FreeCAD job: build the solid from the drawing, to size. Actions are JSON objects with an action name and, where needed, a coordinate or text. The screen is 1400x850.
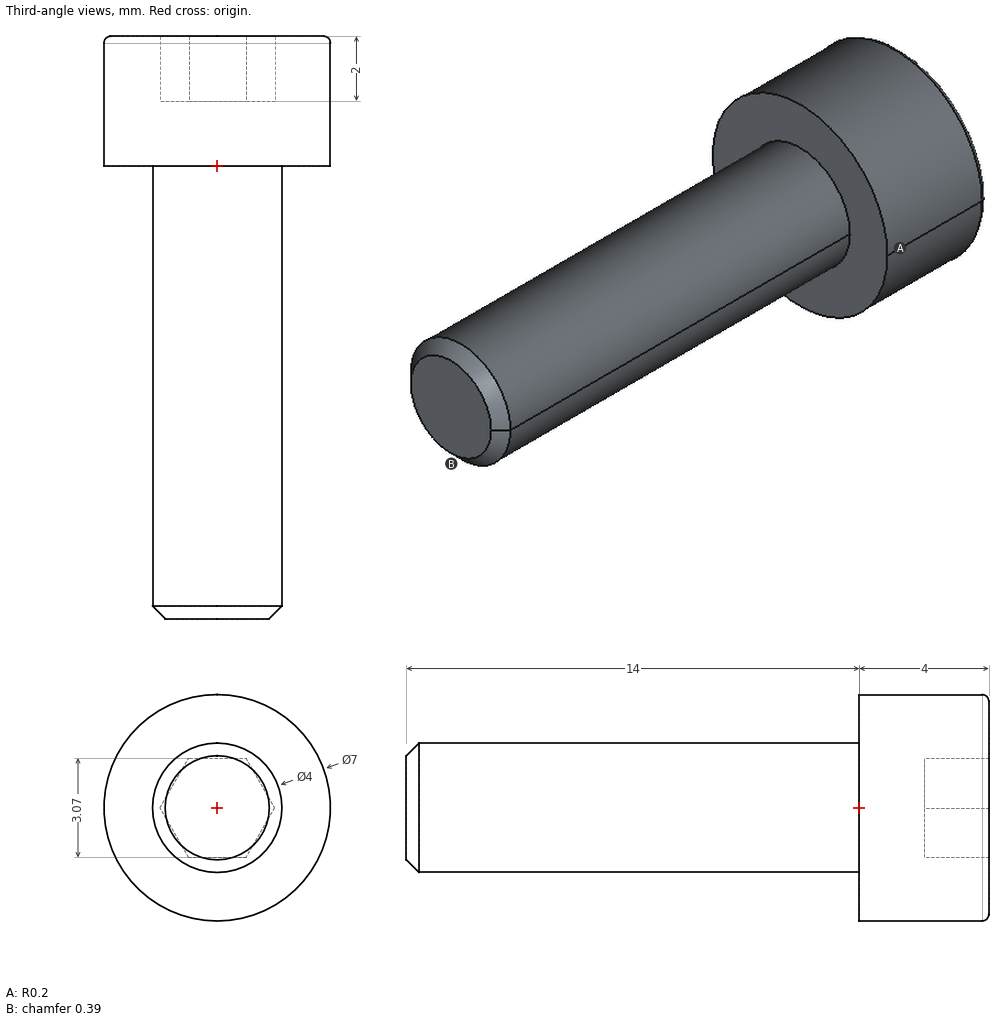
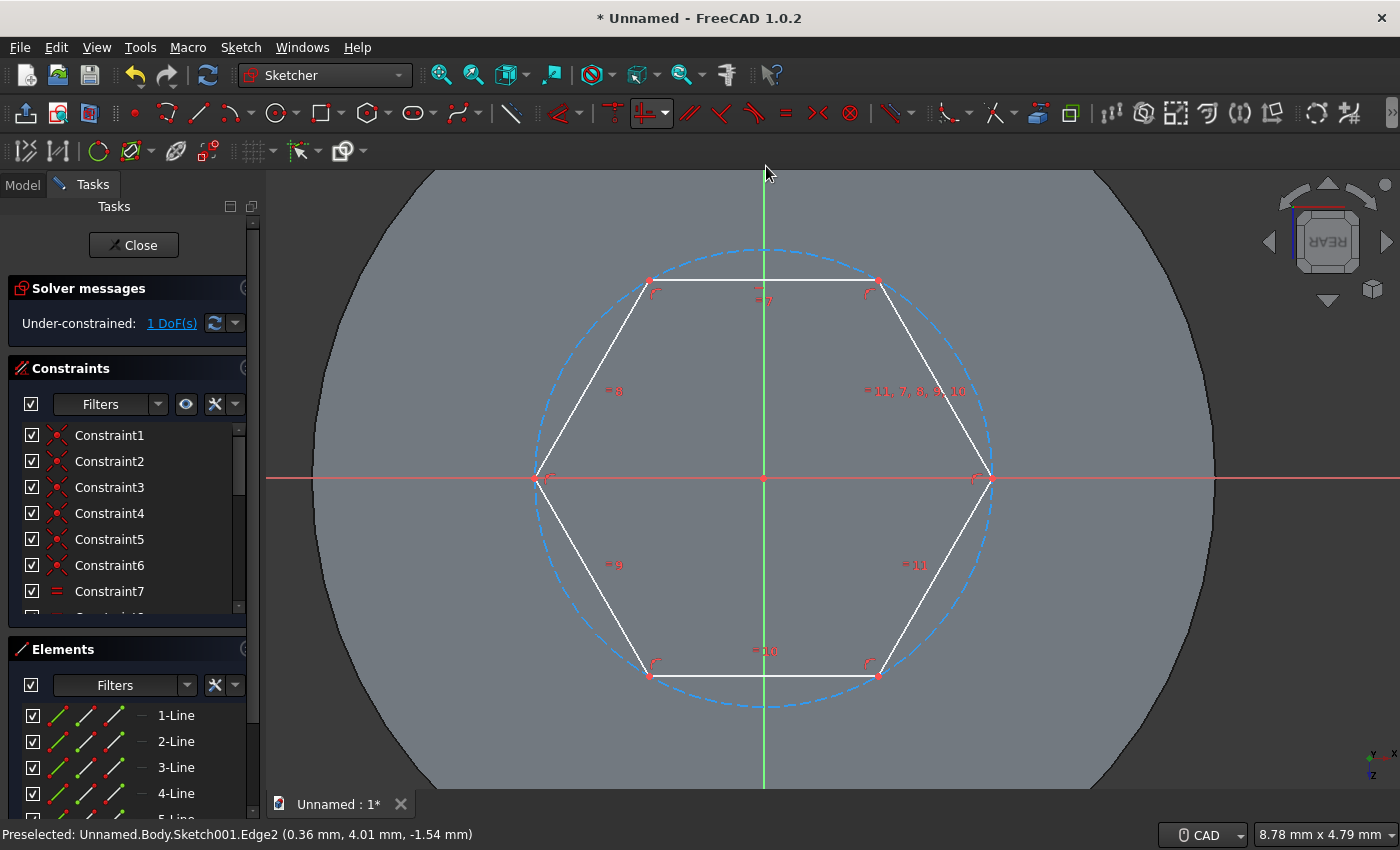
{"action": "left_click", "coordinate": [558, 114]}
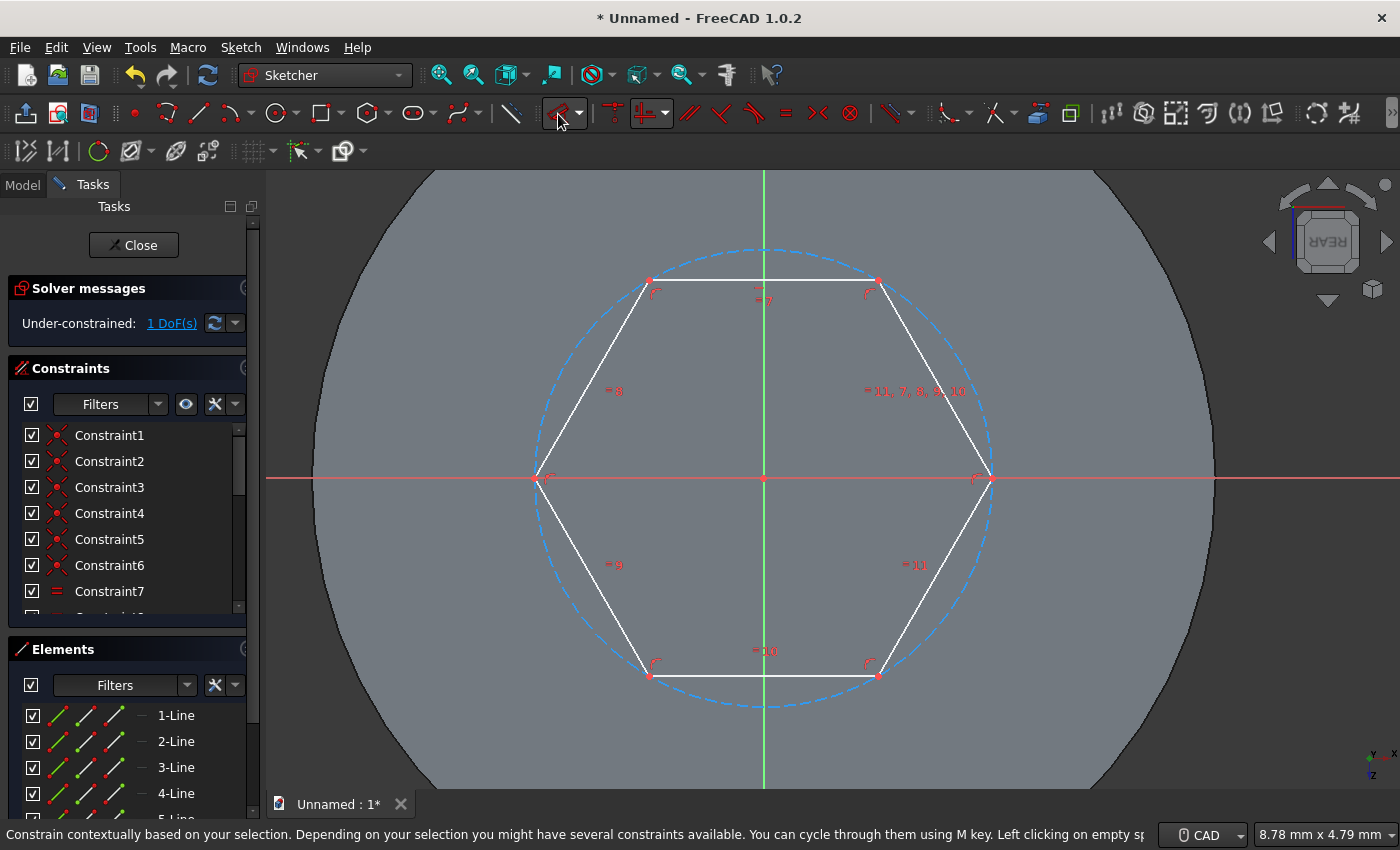
{"action": "left_click", "coordinate": [649, 676]}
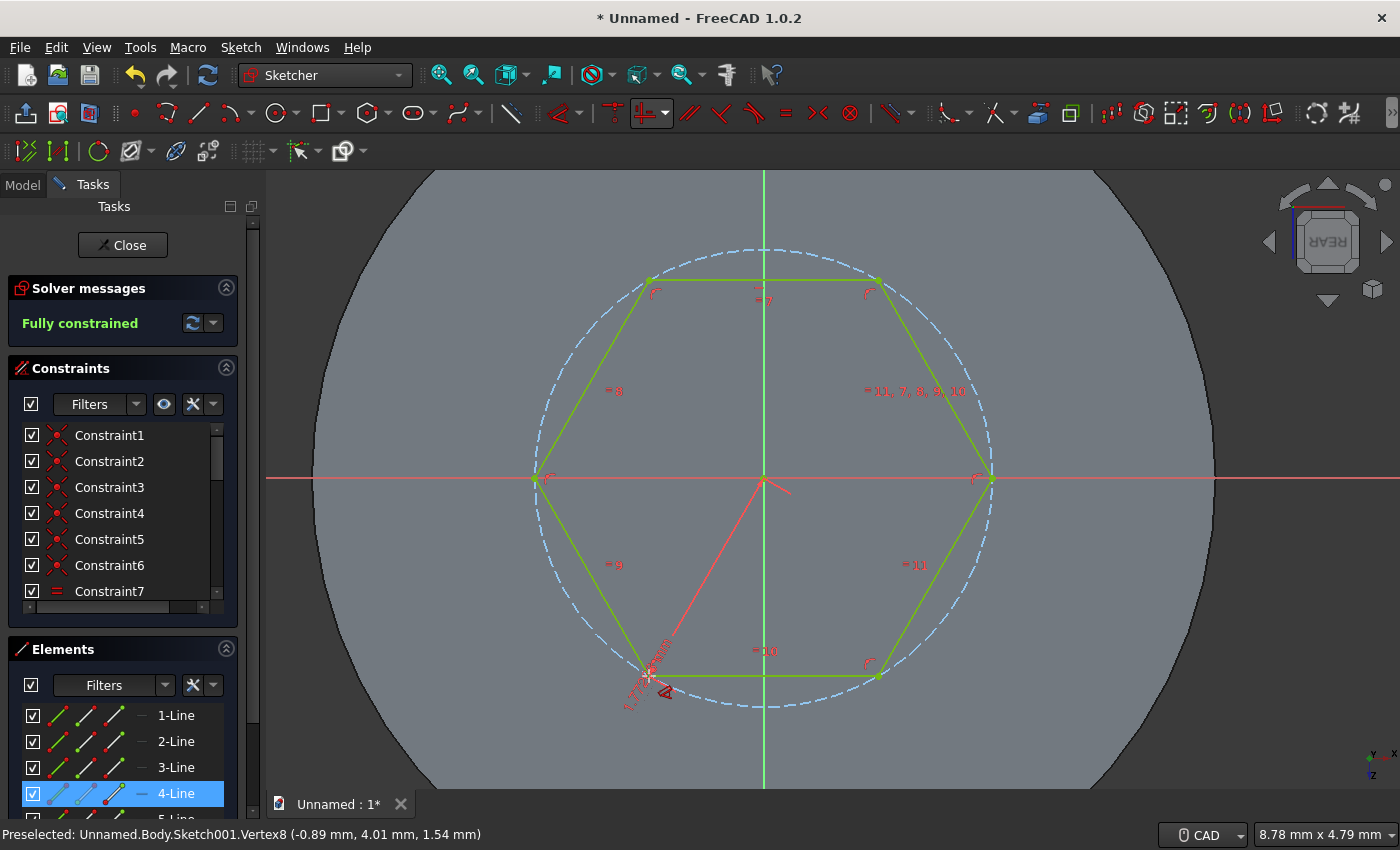
{"action": "left_click", "coordinate": [878, 280]}
{"action": "left_click", "coordinate": [615, 387]}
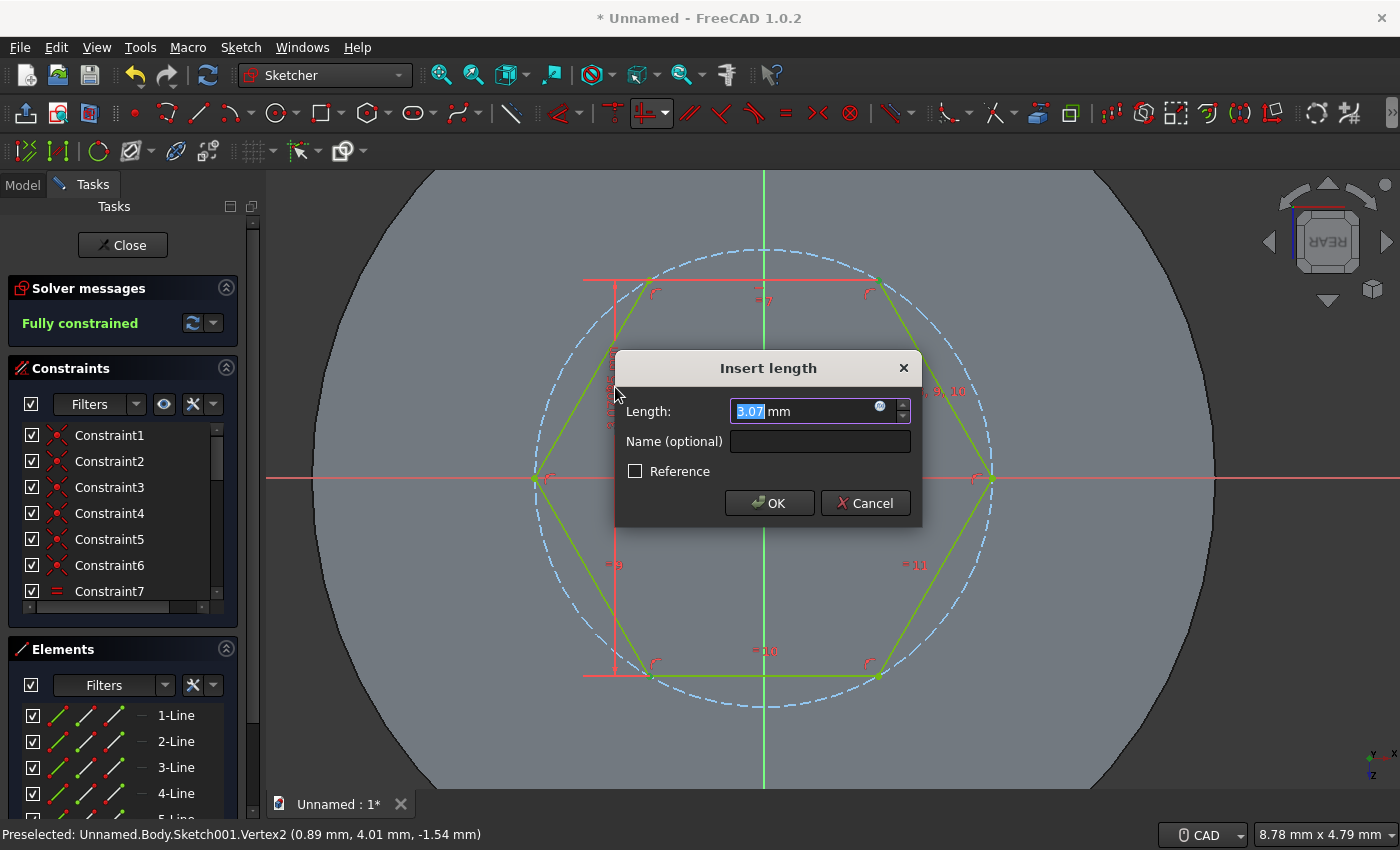
{"action": "type", "text": "3.07"}
{"action": "key", "text": "Return"}
{"action": "key", "text": "Escape"}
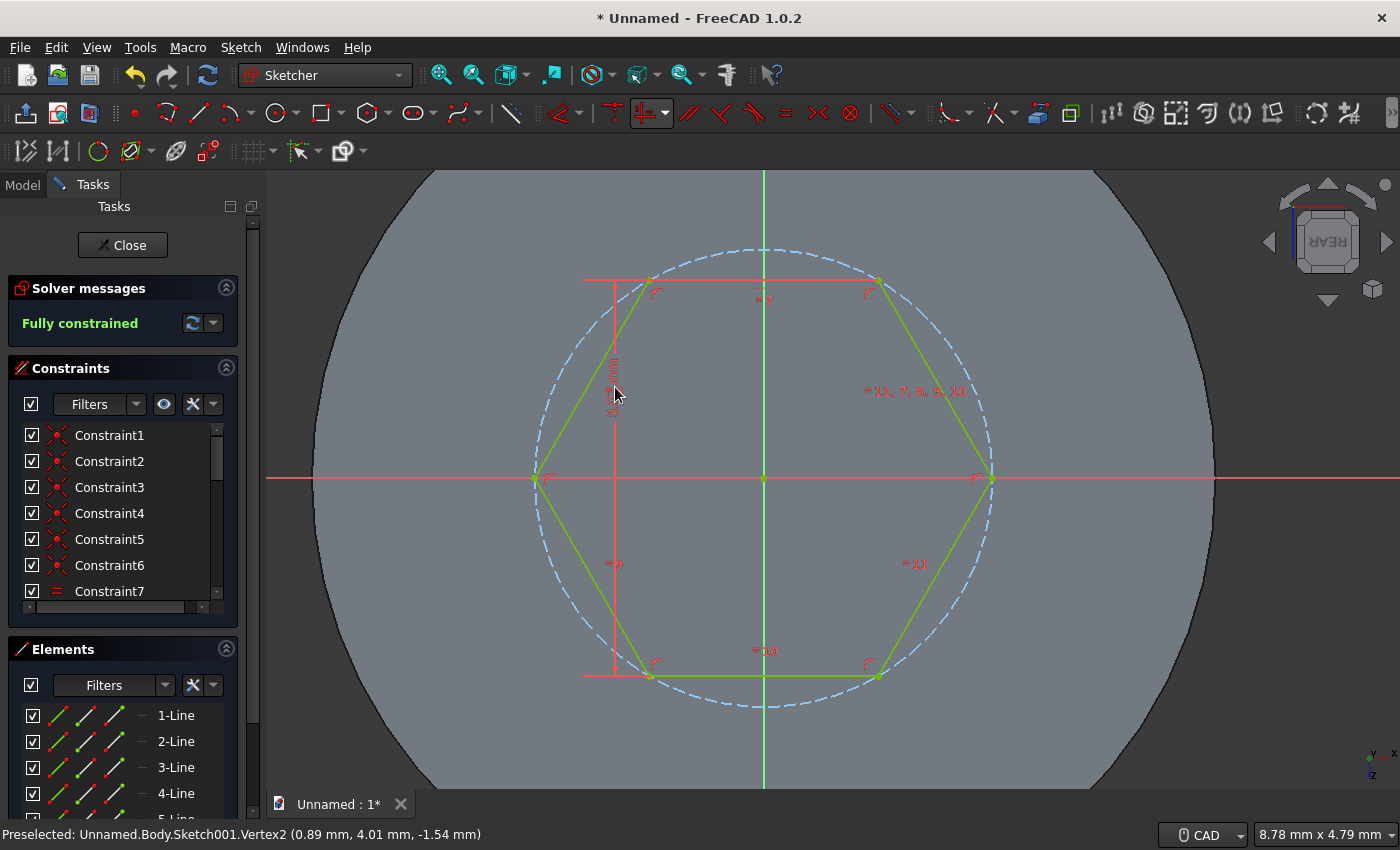
{"action": "left_click", "coordinate": [123, 245]}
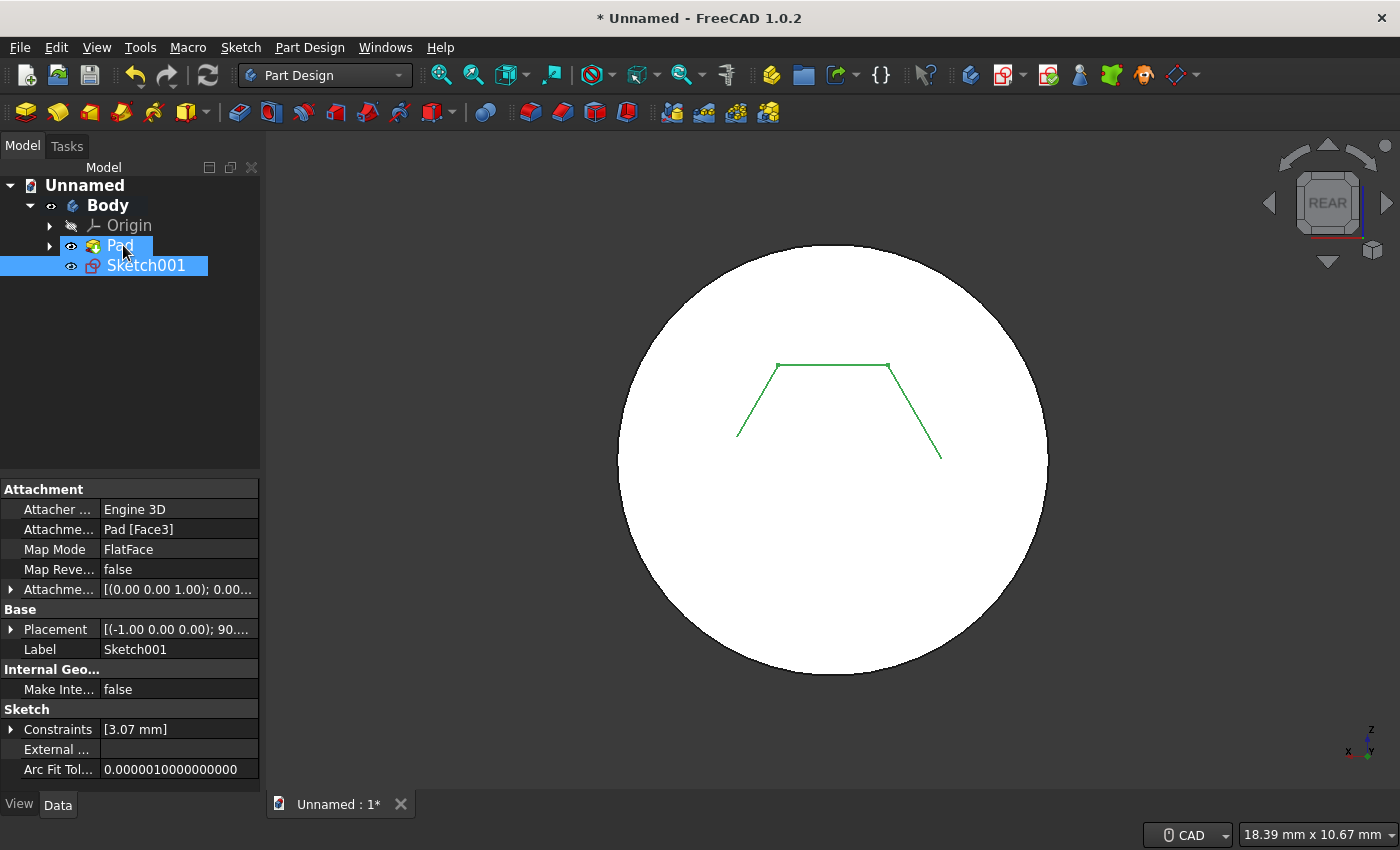
{"action": "left_click", "coordinate": [240, 112]}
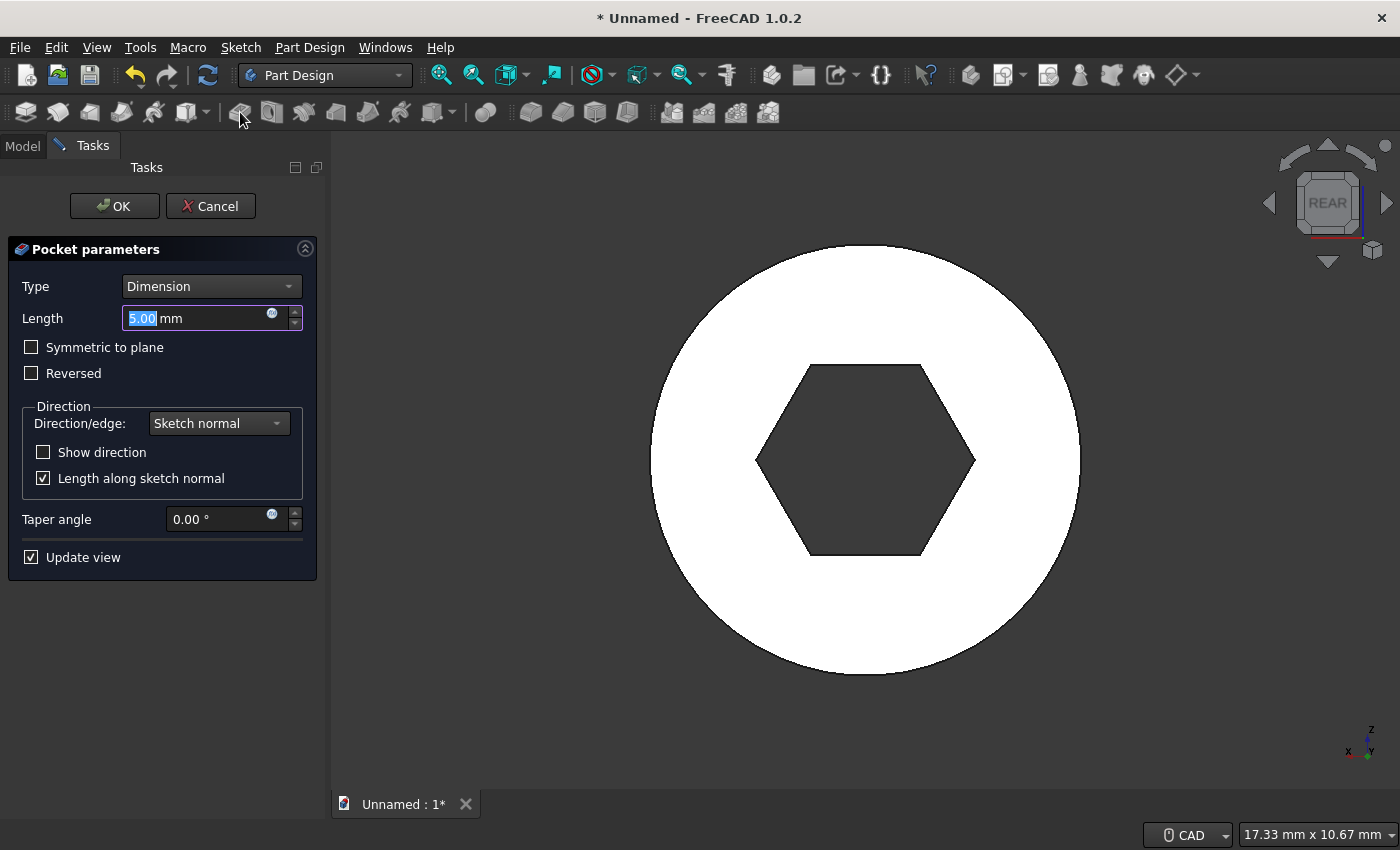
{"action": "type", "text": "2"}
{"action": "key", "text": "Tab"}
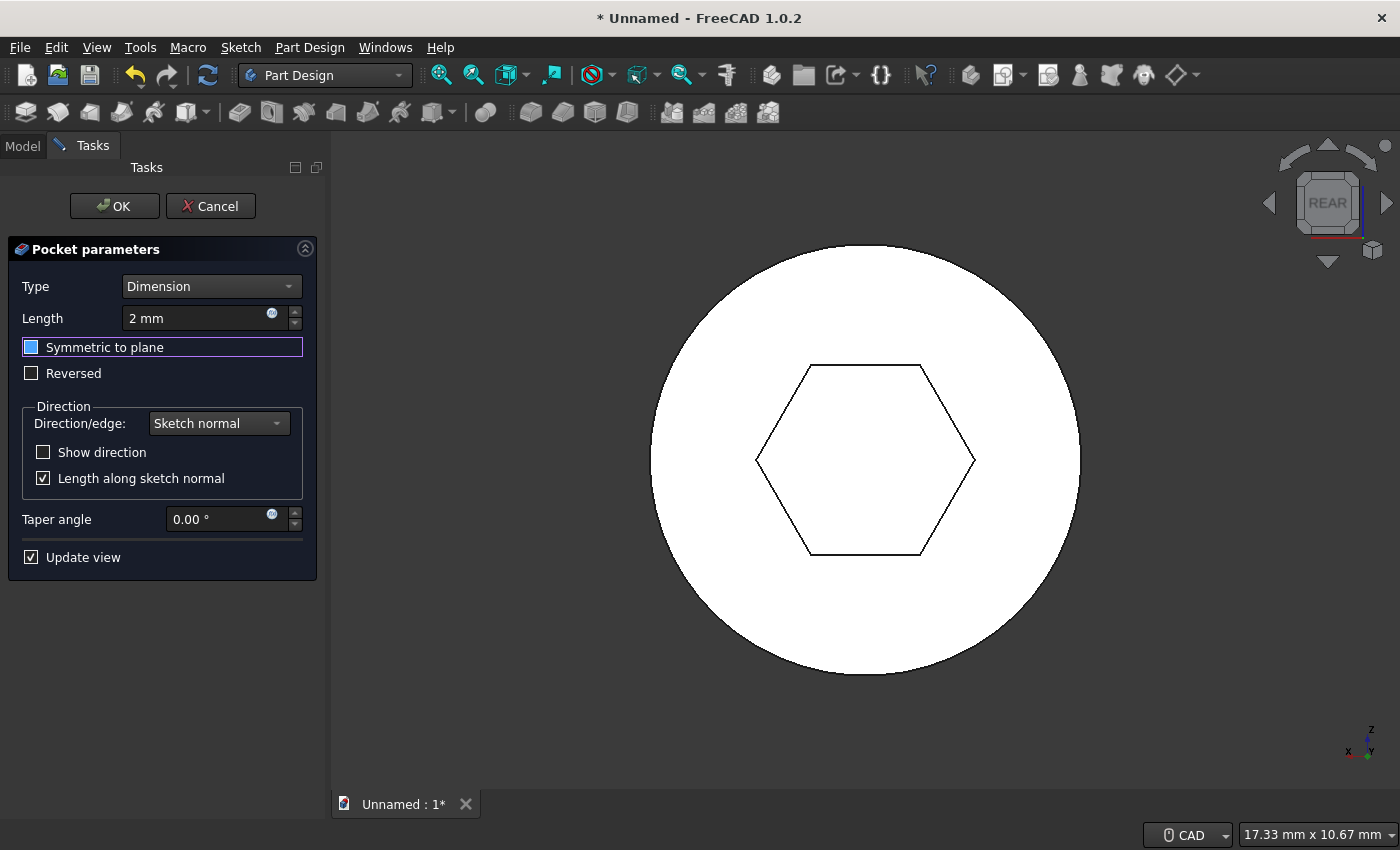
{"action": "left_click", "coordinate": [115, 206]}